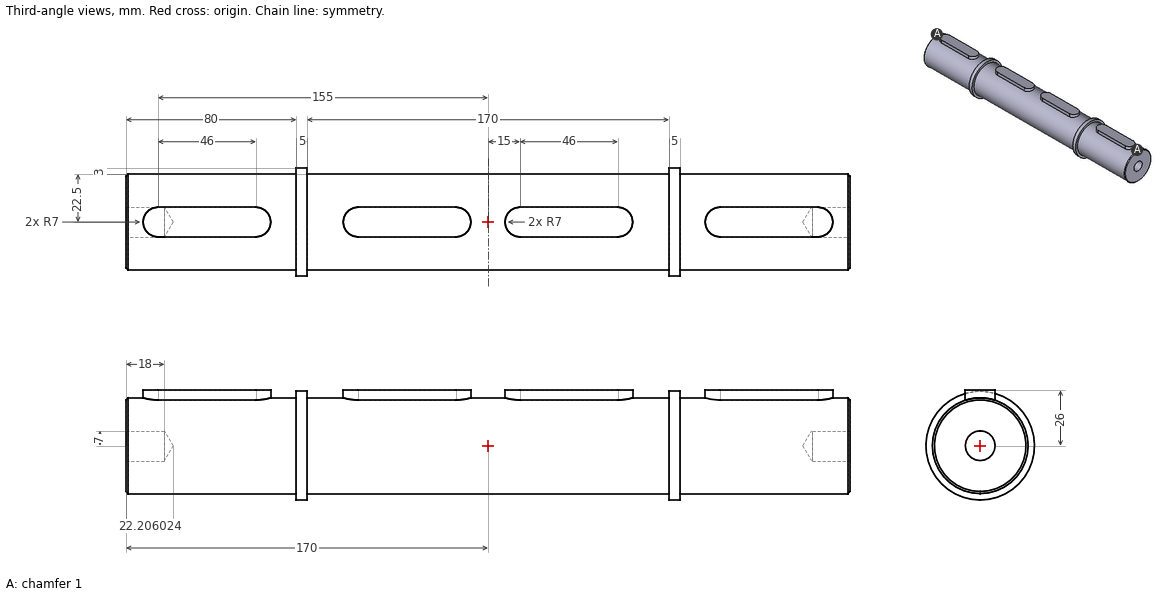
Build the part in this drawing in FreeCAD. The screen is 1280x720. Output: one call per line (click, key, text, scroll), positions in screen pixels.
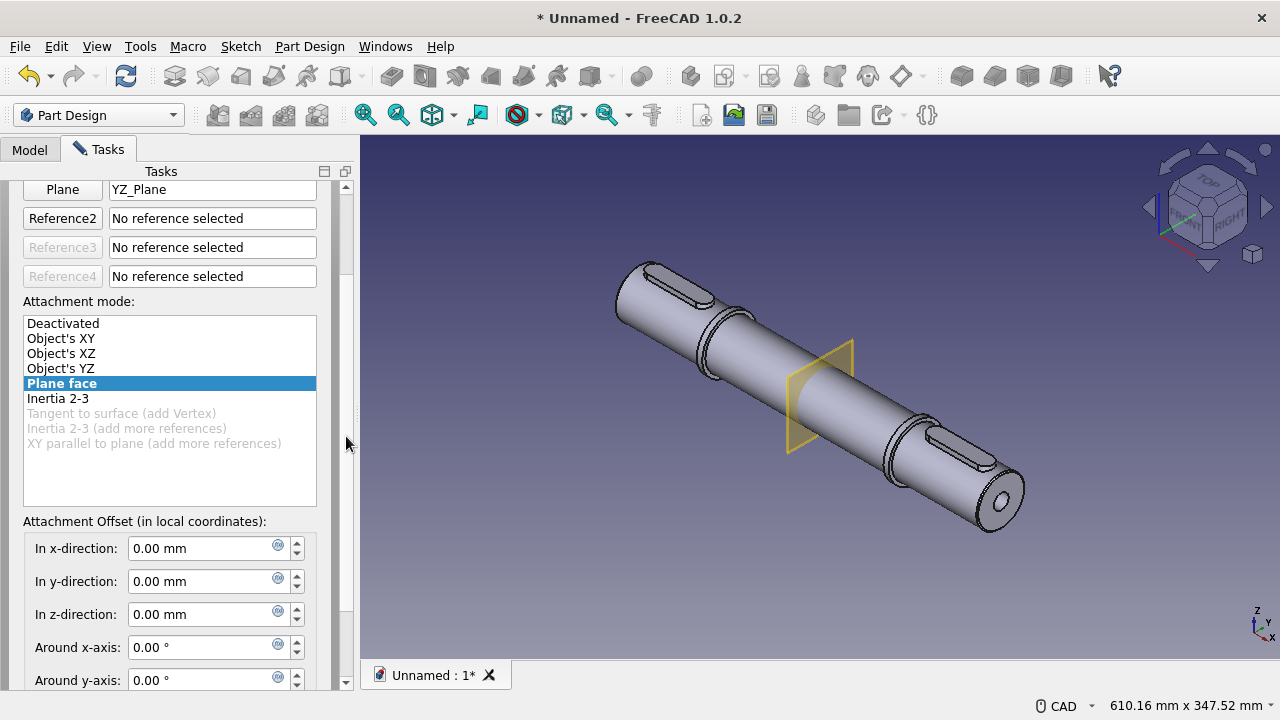
triple_click(210, 614)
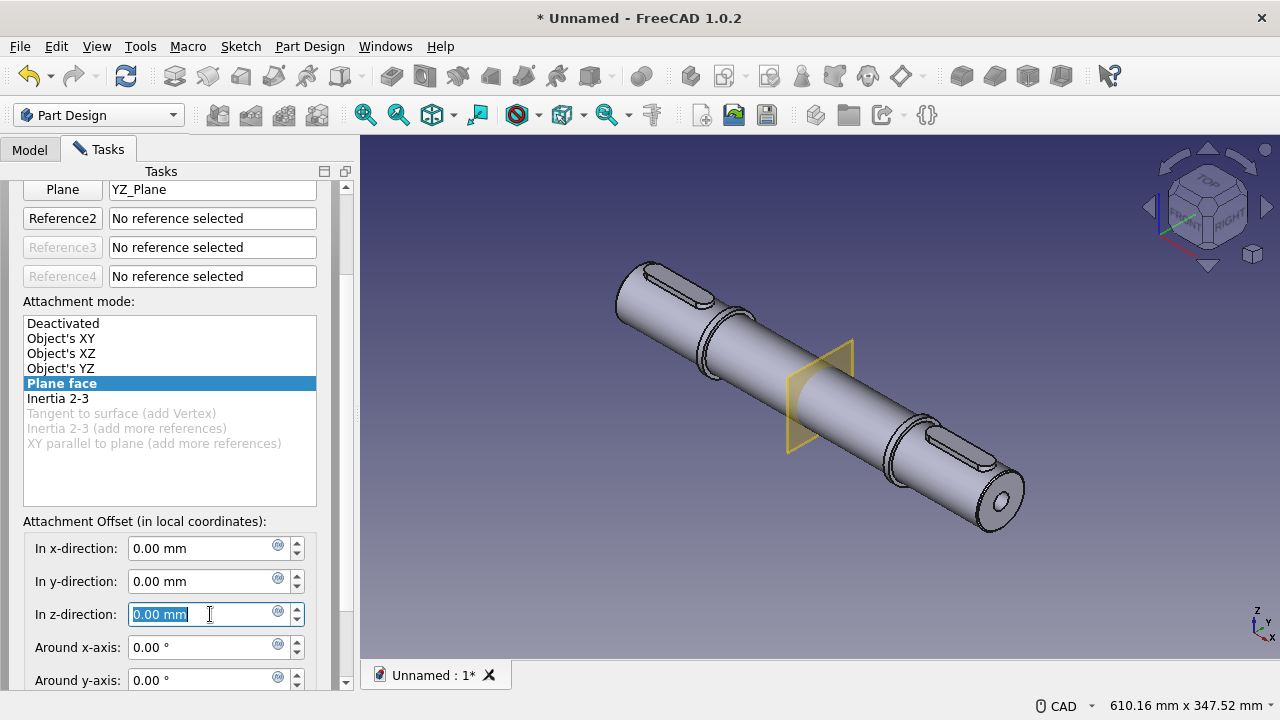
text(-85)
key(Tab)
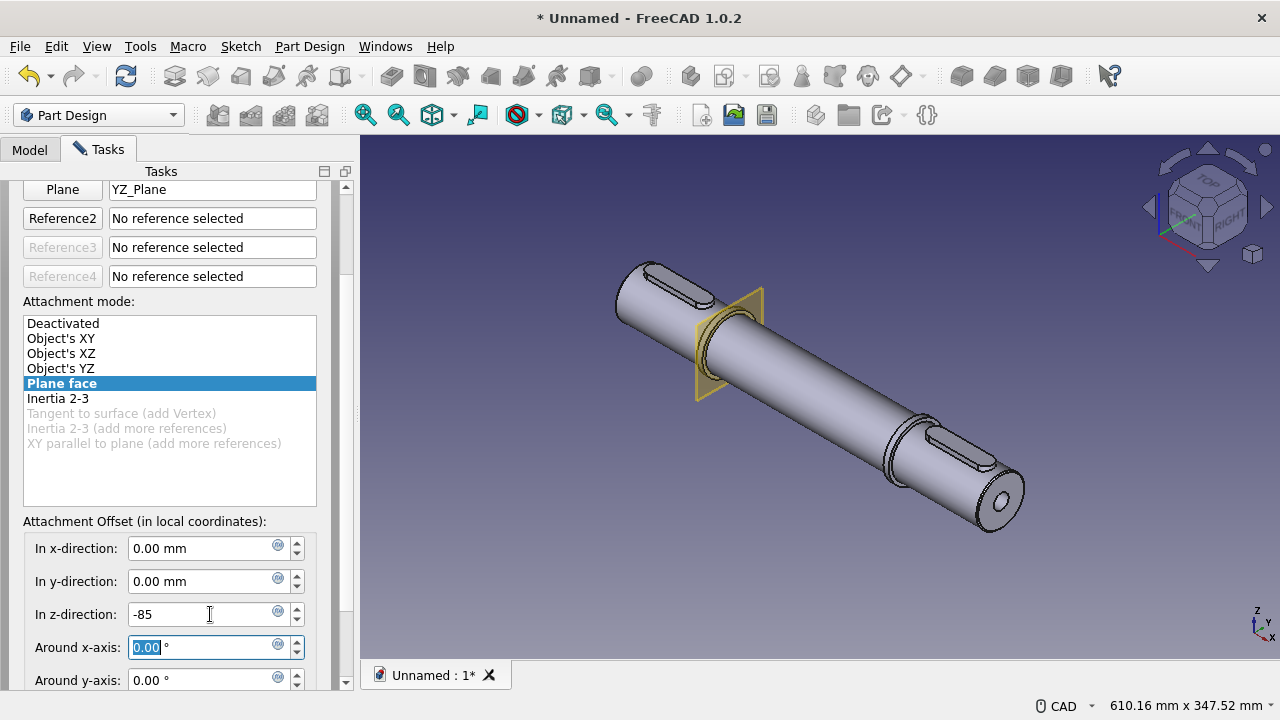
scroll(346, 436, up, 3)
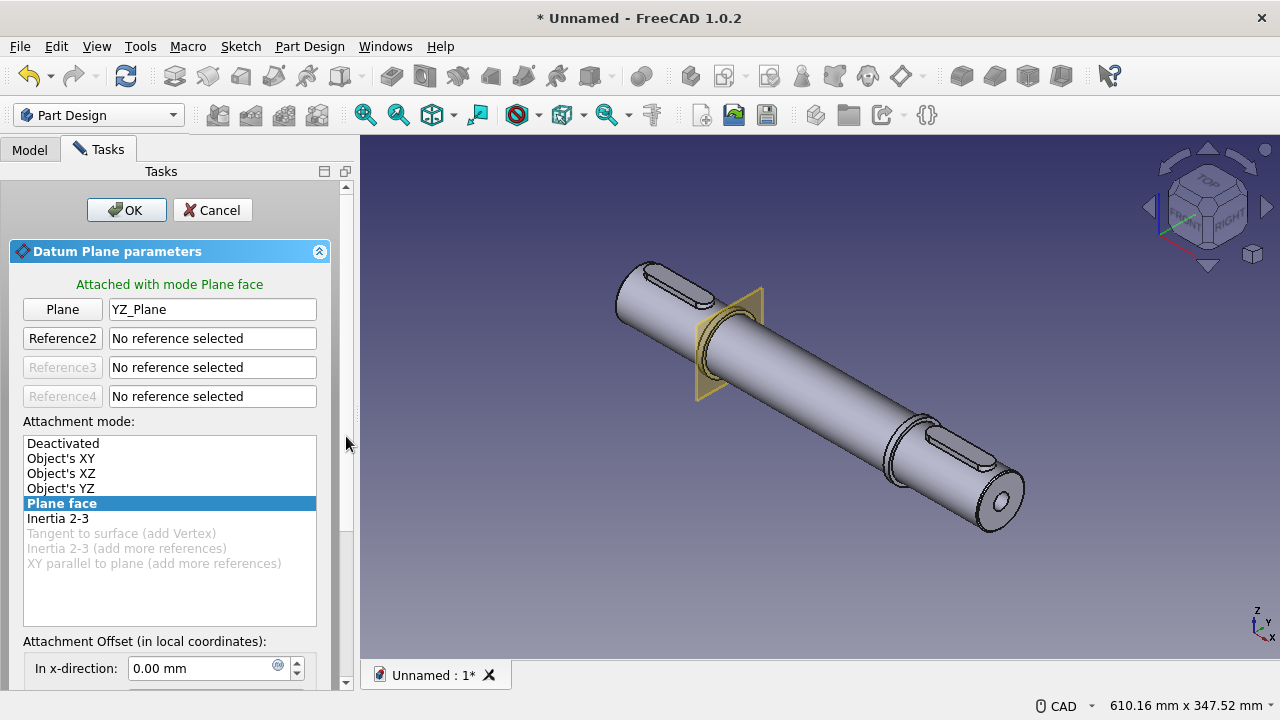
click(127, 210)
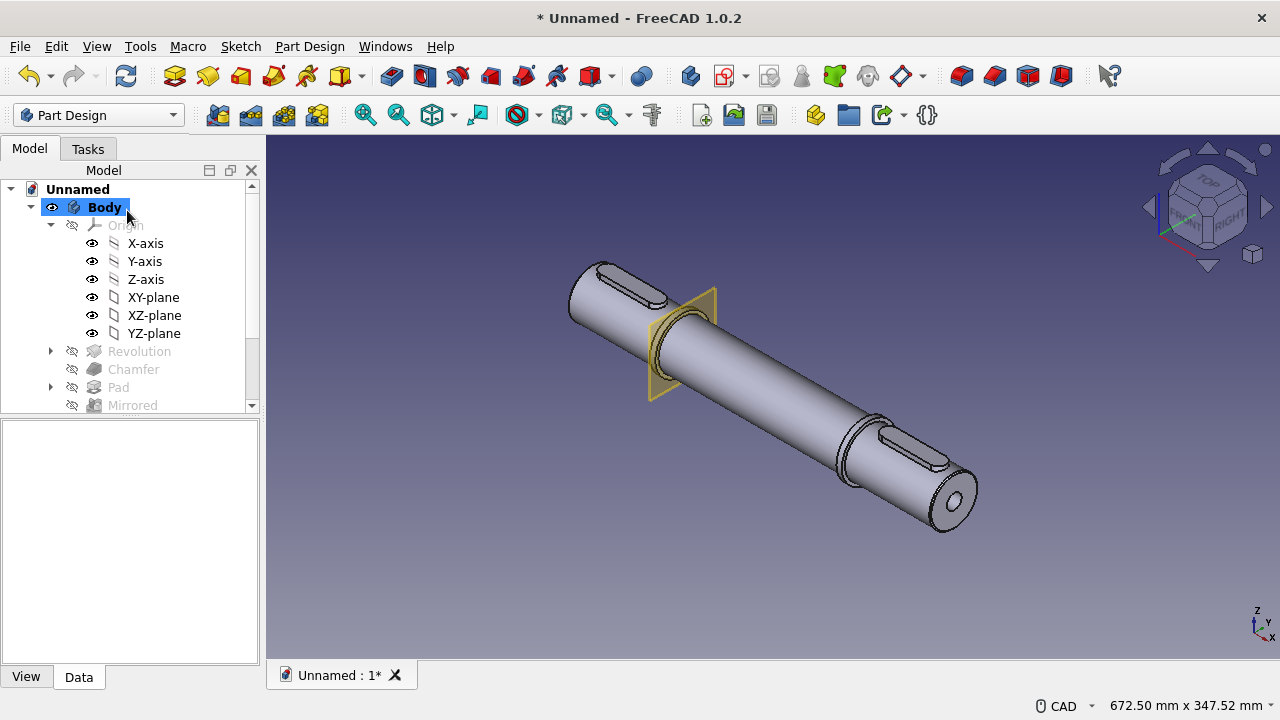
click(117, 387)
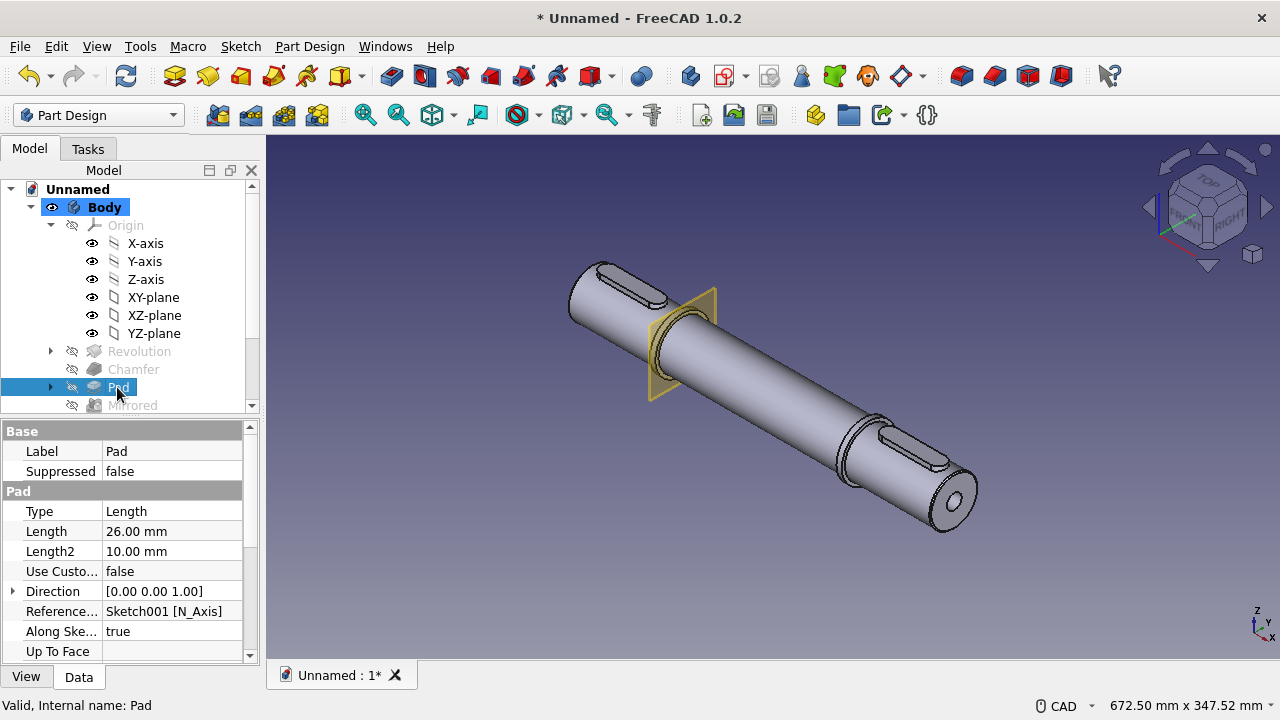
click(218, 116)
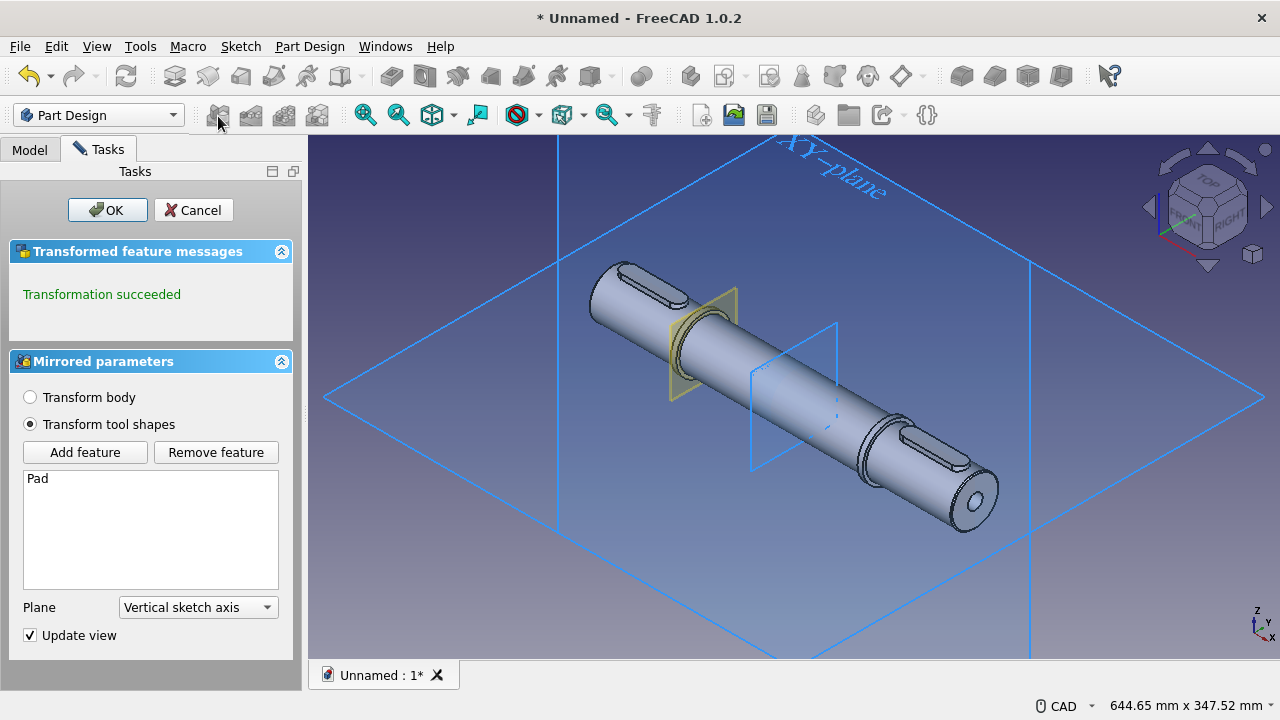
click(199, 608)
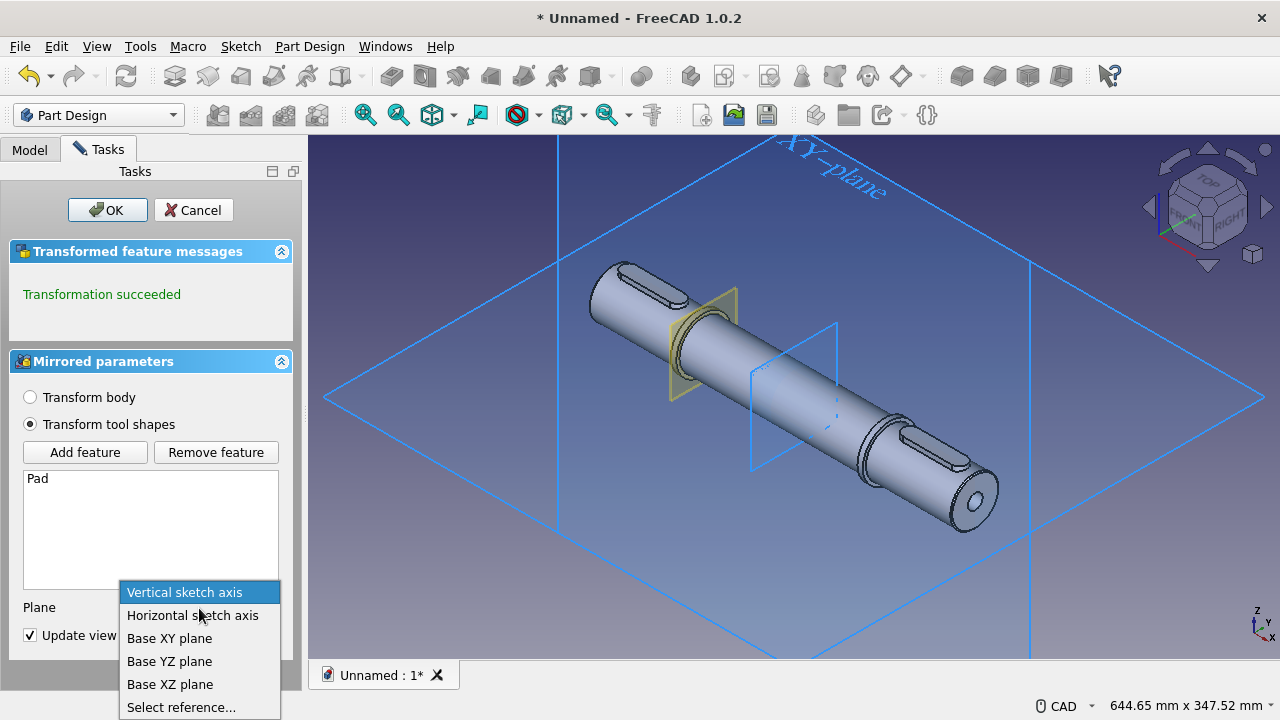
click(198, 708)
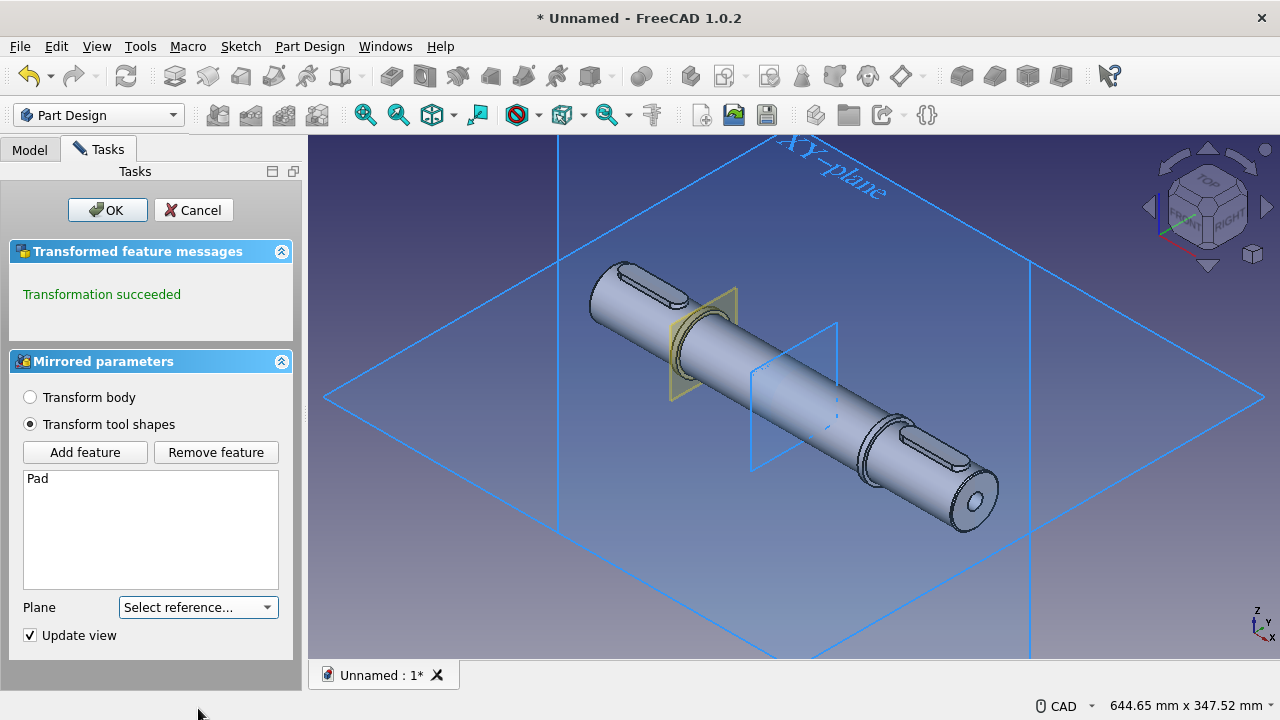
click(30, 149)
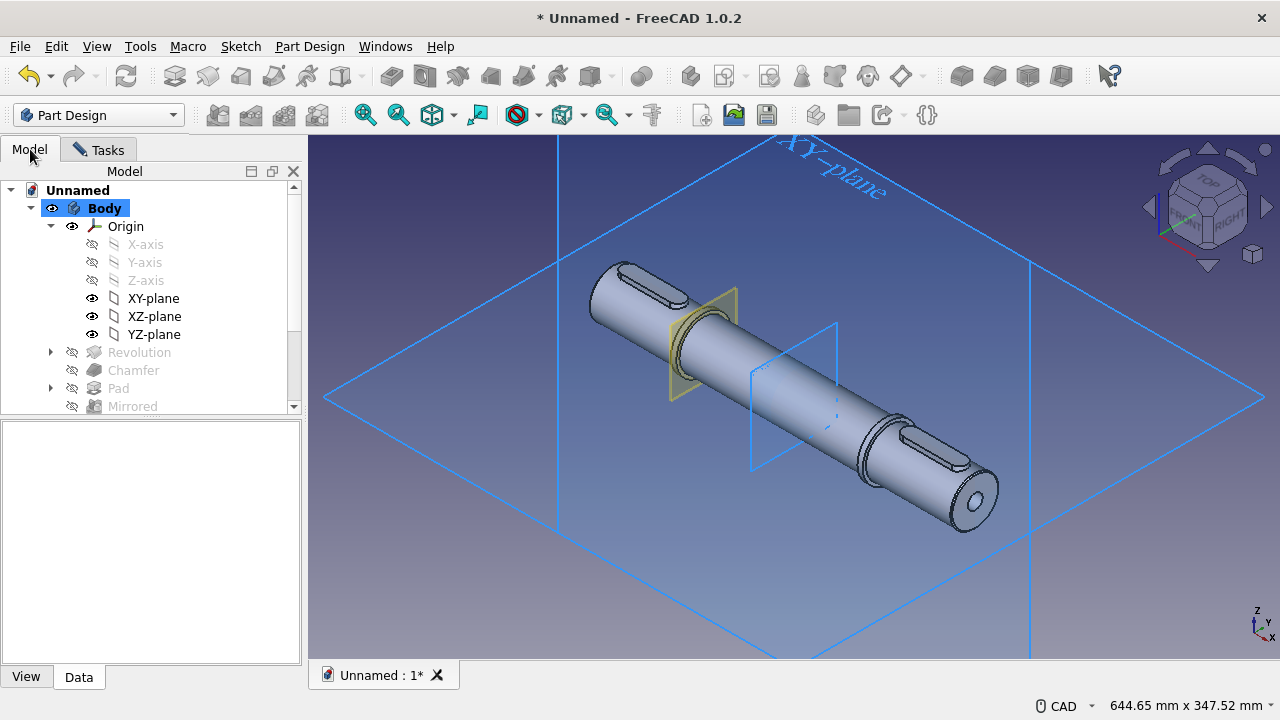
scroll(101, 294, down, 3)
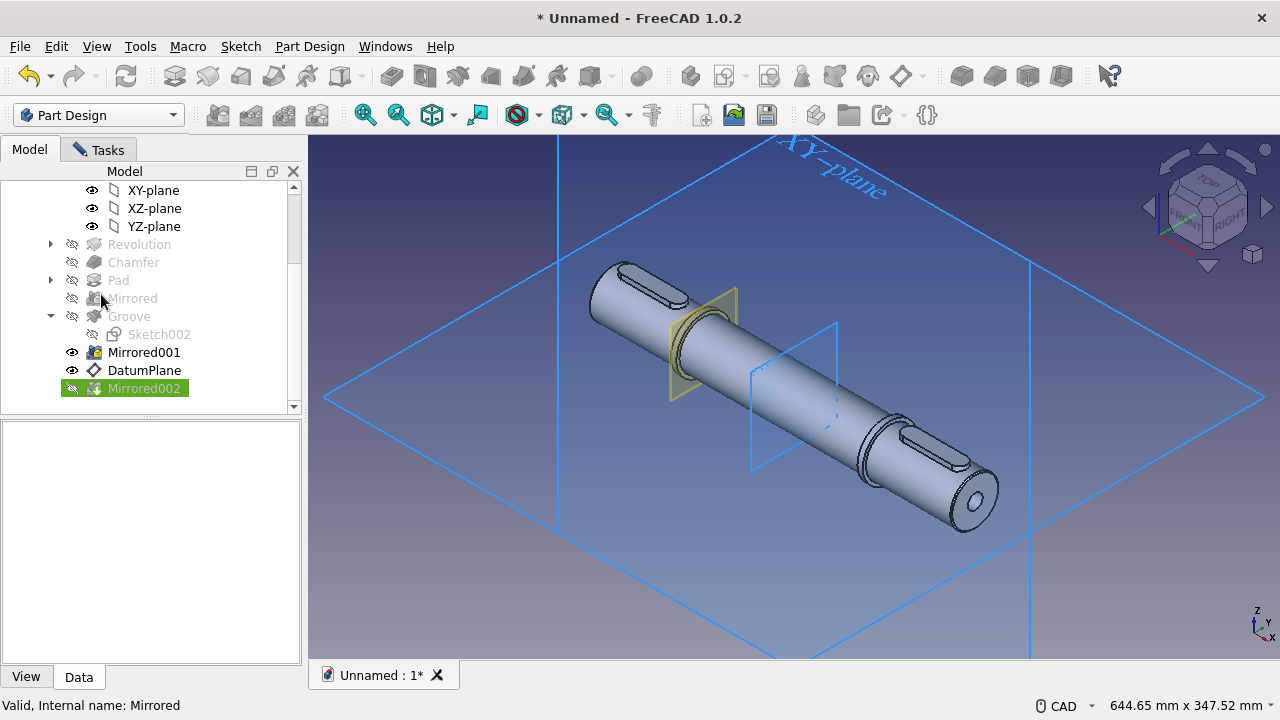
click(117, 370)